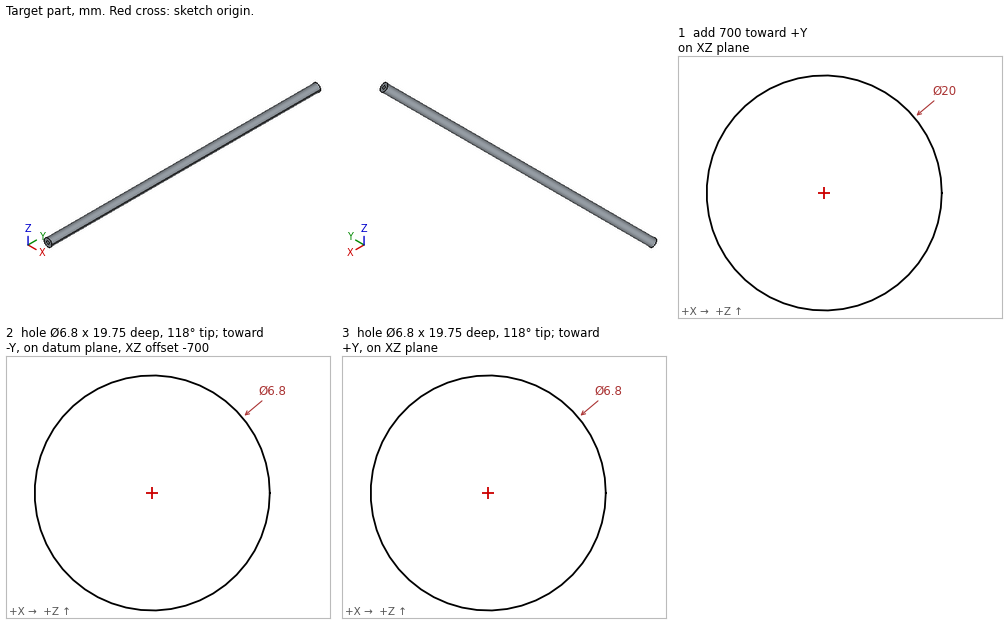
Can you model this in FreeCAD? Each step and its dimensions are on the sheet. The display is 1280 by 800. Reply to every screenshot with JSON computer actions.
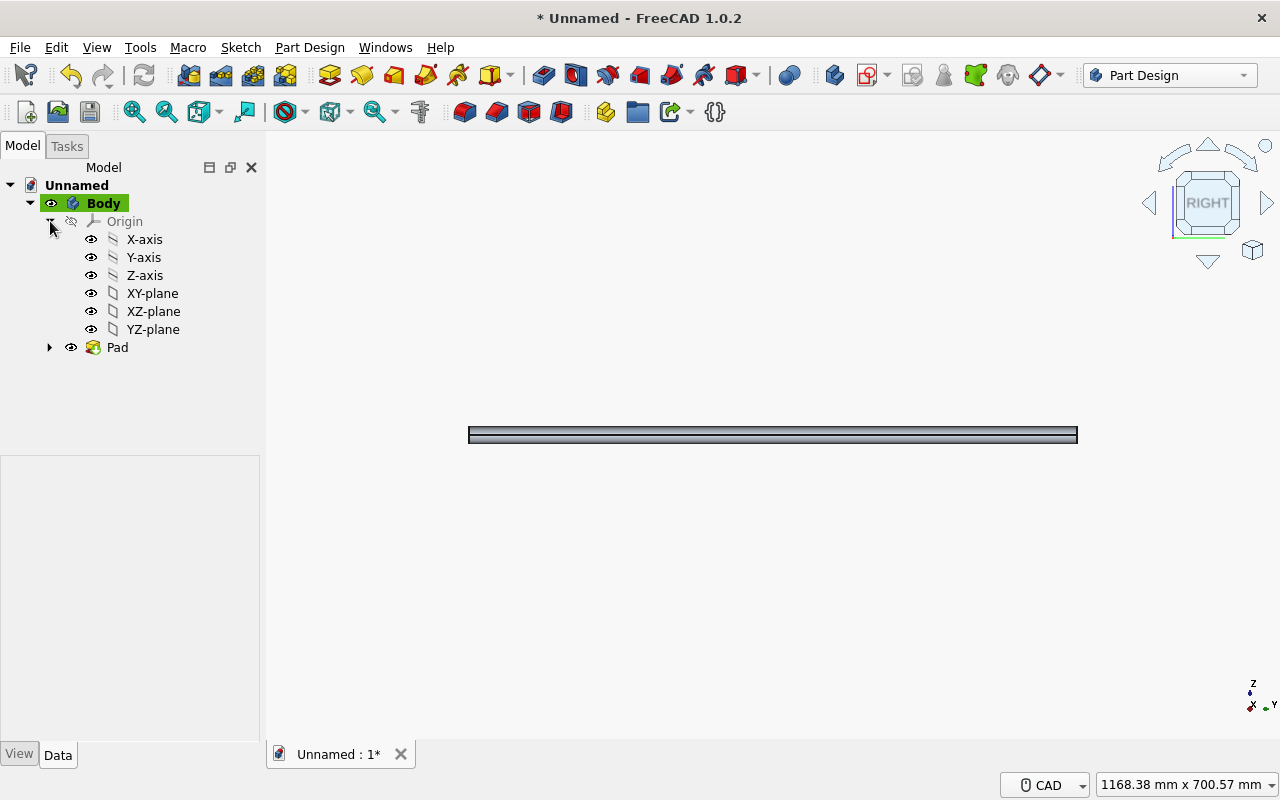
{"action": "left_click", "coordinate": [136, 311]}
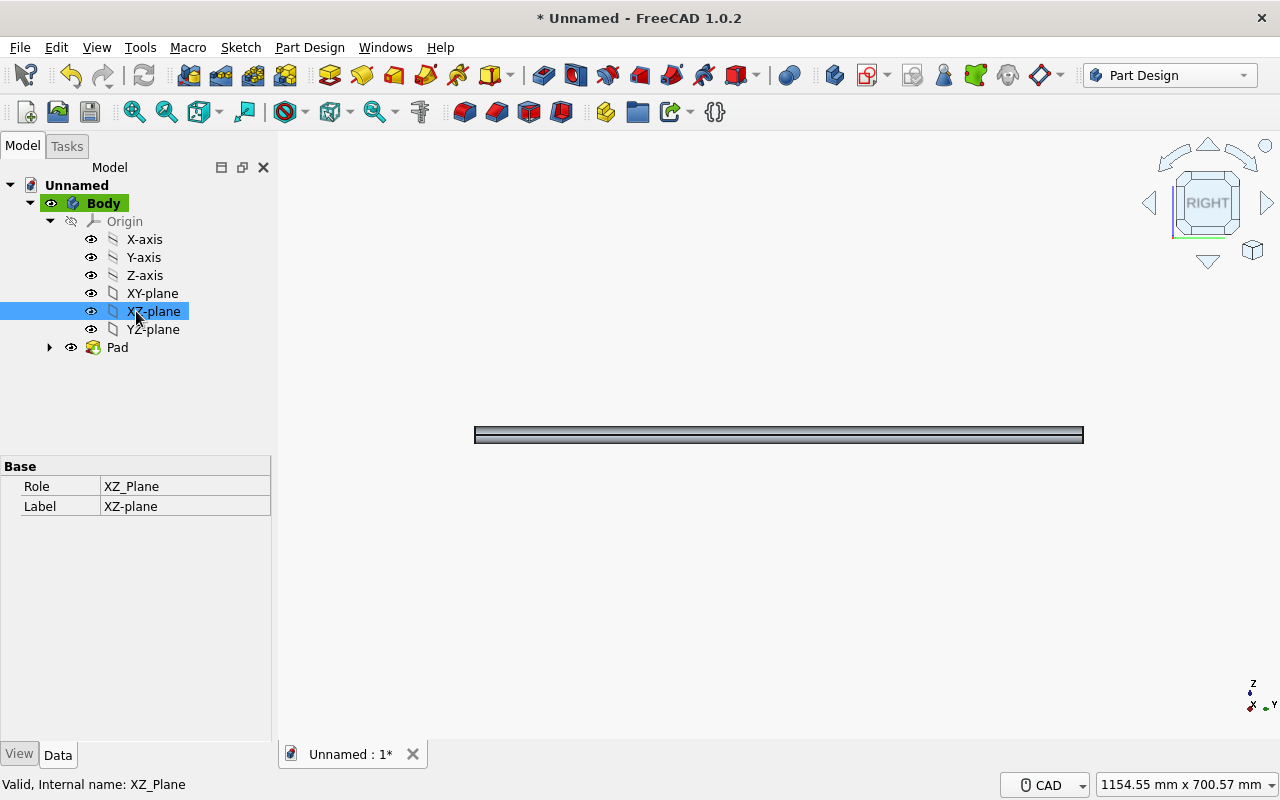
{"action": "left_click", "coordinate": [1040, 76]}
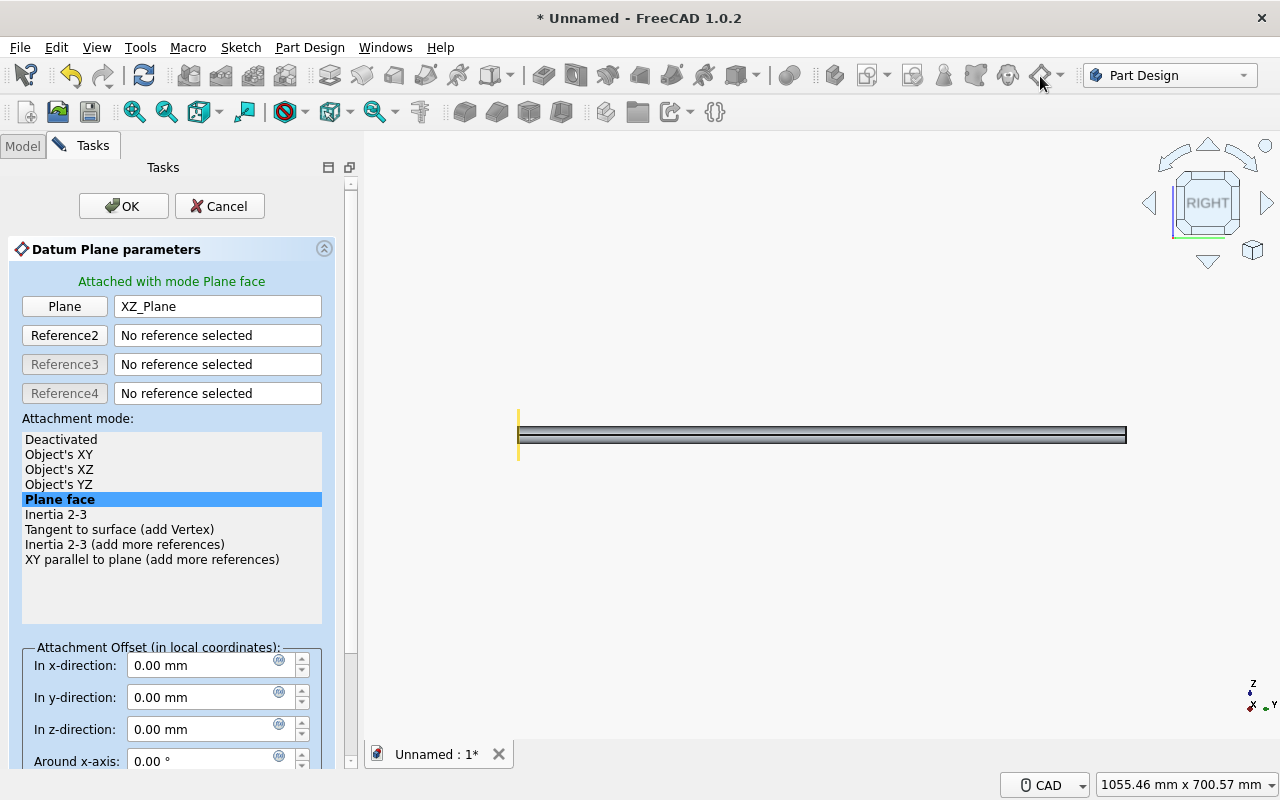
{"action": "triple_click", "coordinate": [210, 729]}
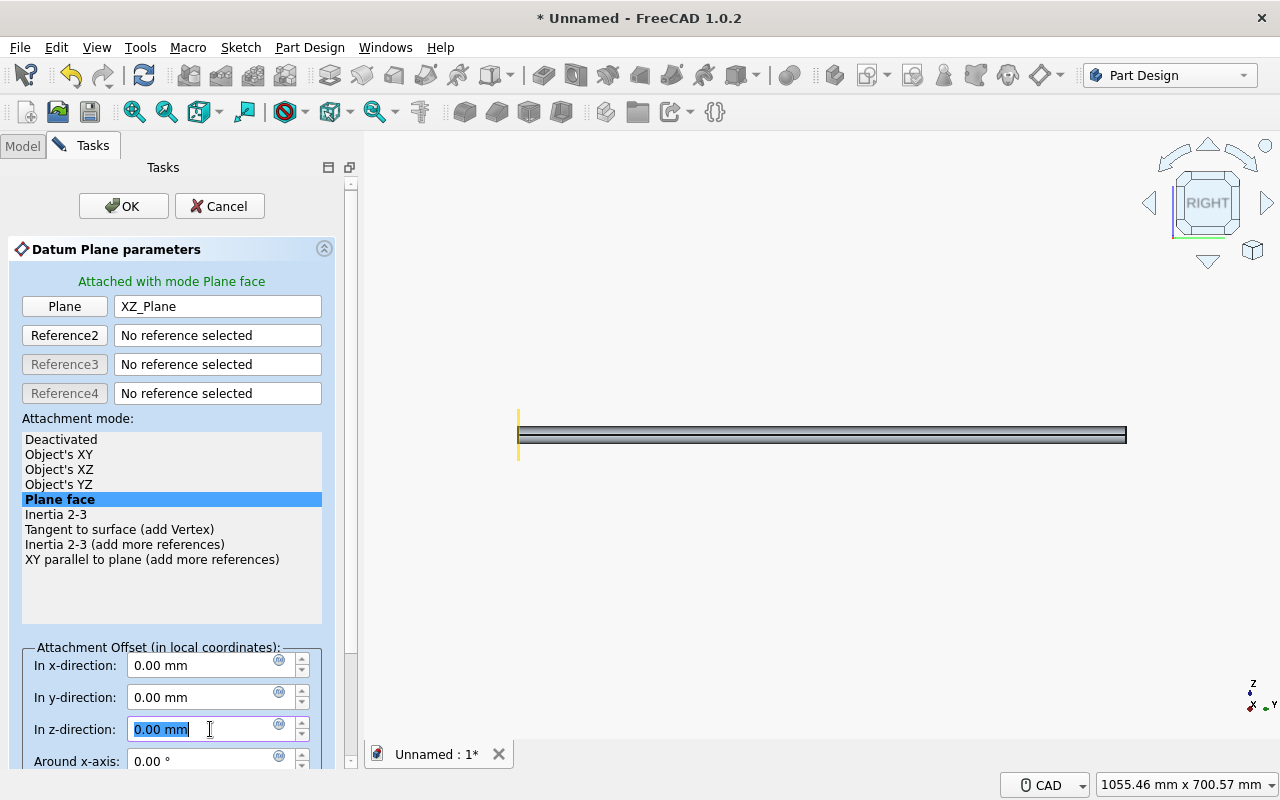
{"action": "type", "text": "-700"}
{"action": "key", "text": "Tab"}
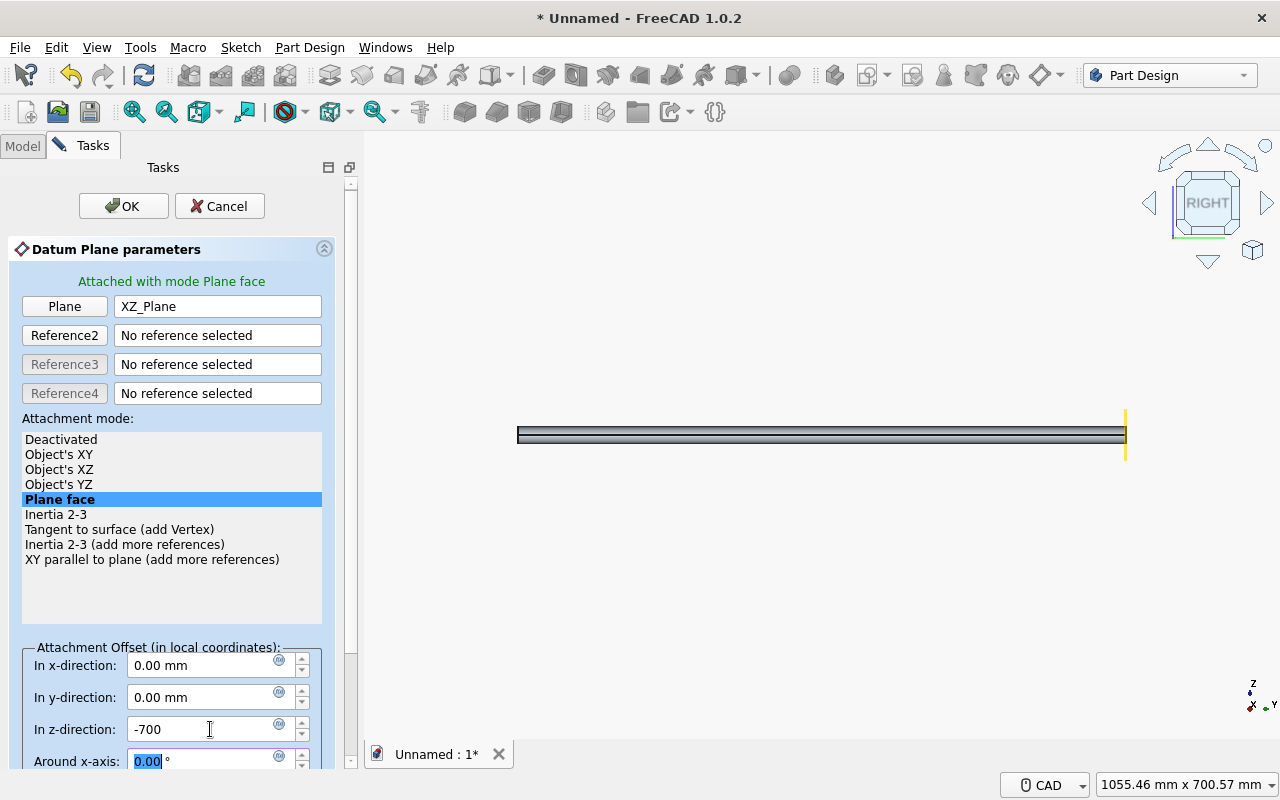
{"action": "left_click", "coordinate": [124, 206]}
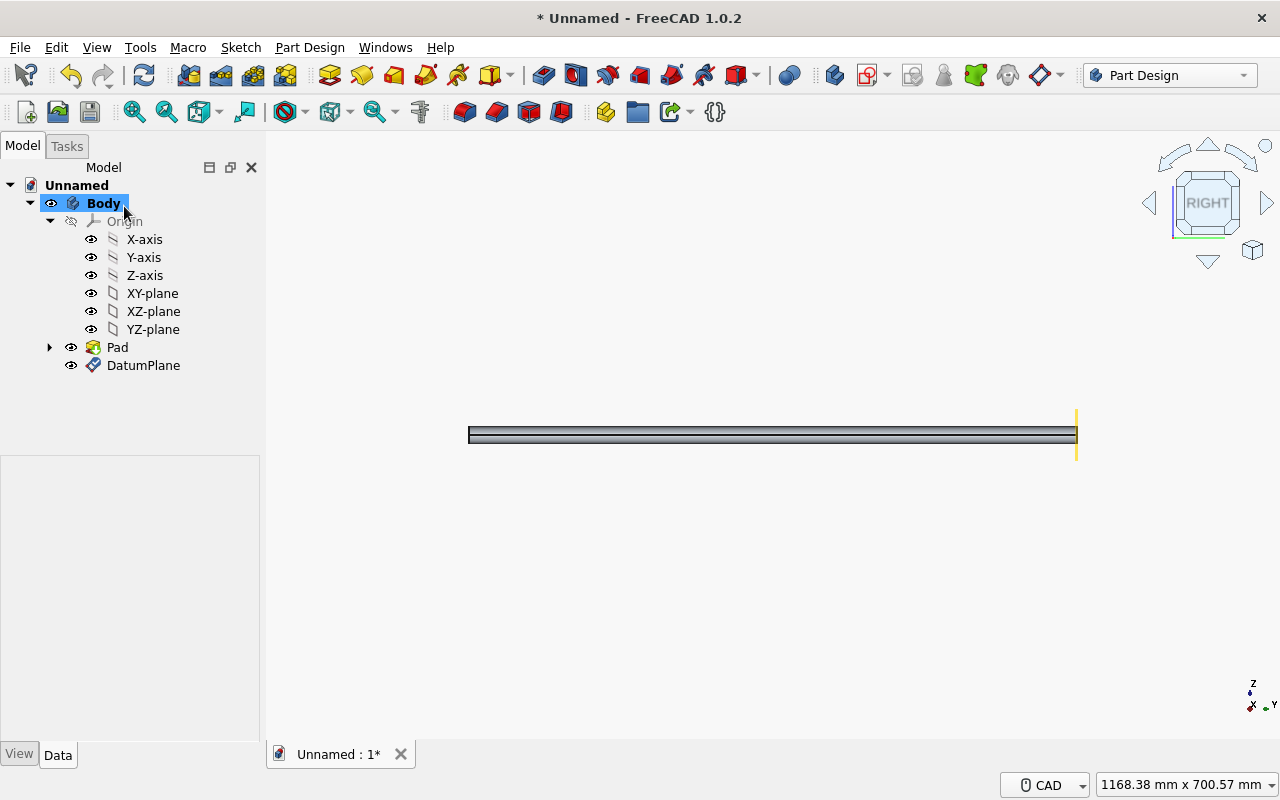
{"action": "left_click", "coordinate": [116, 365]}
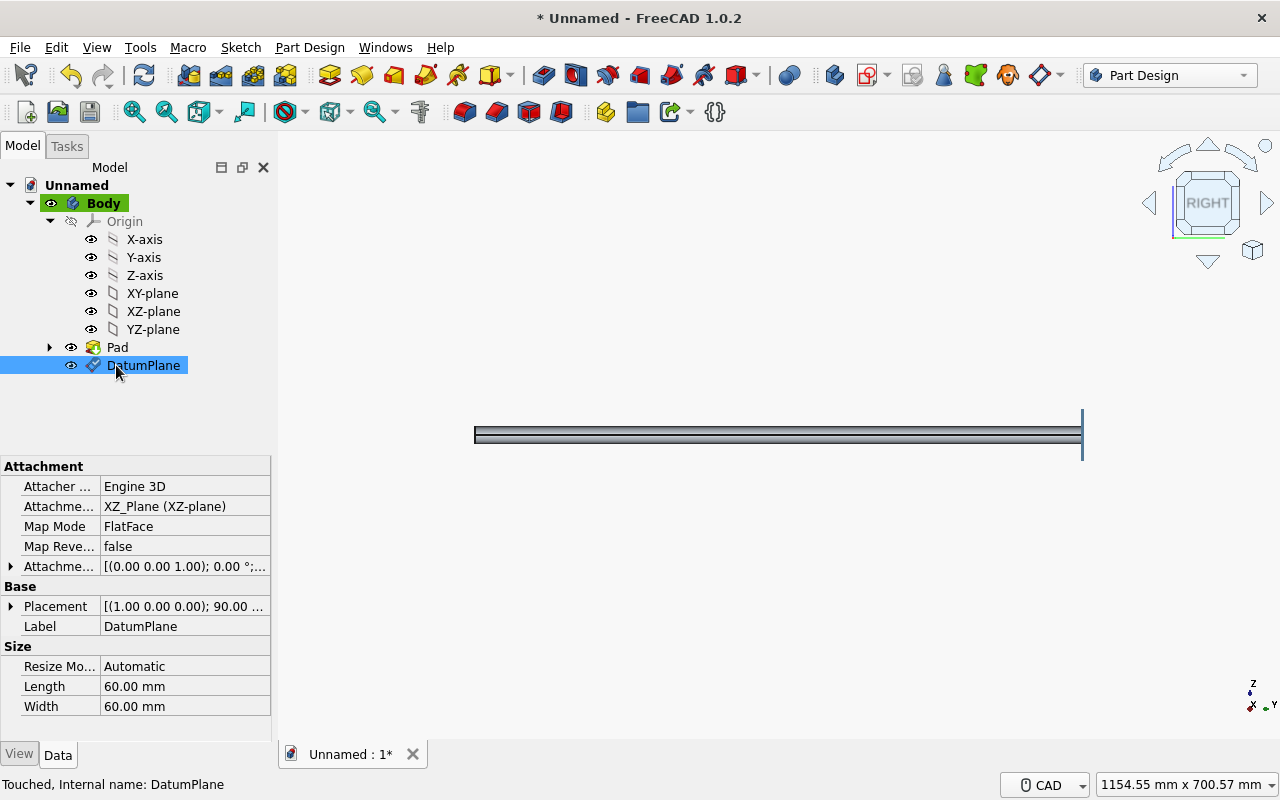
{"action": "left_click", "coordinate": [868, 76]}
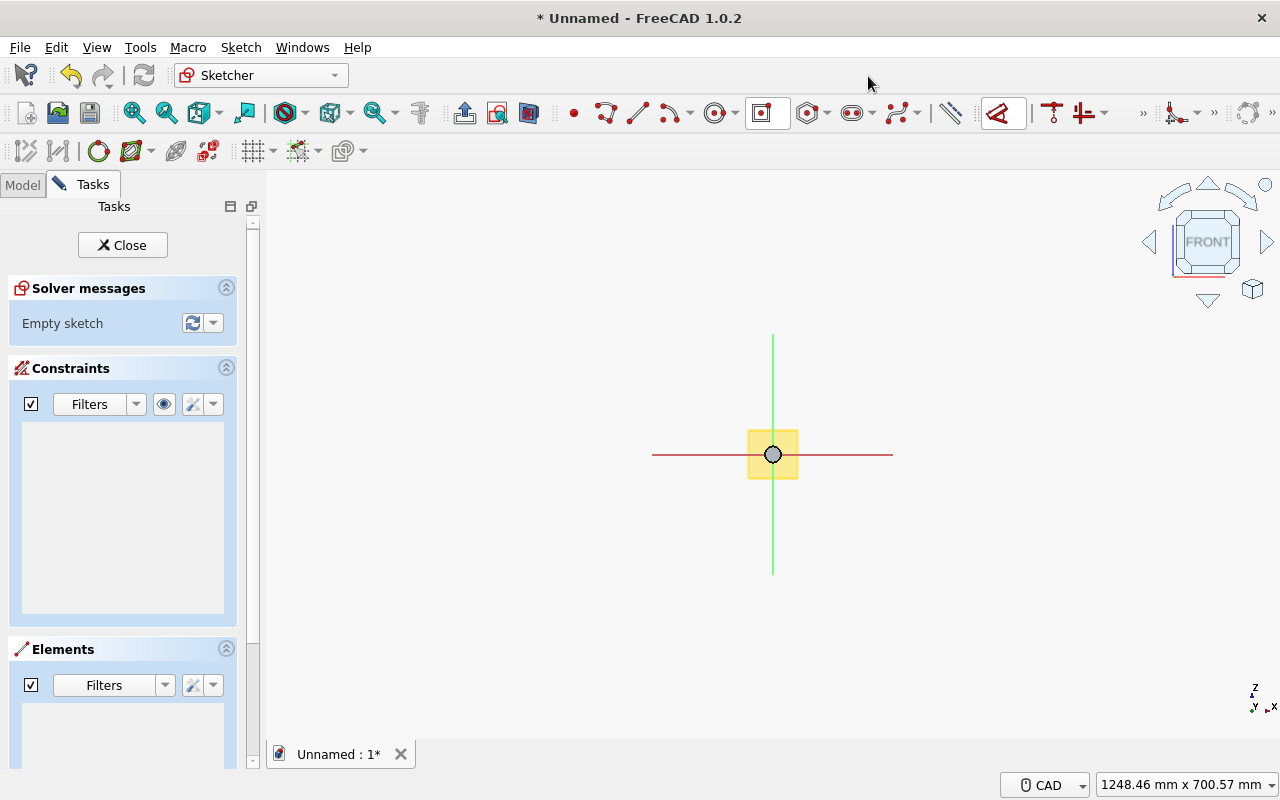
{"action": "left_click", "coordinate": [530, 114]}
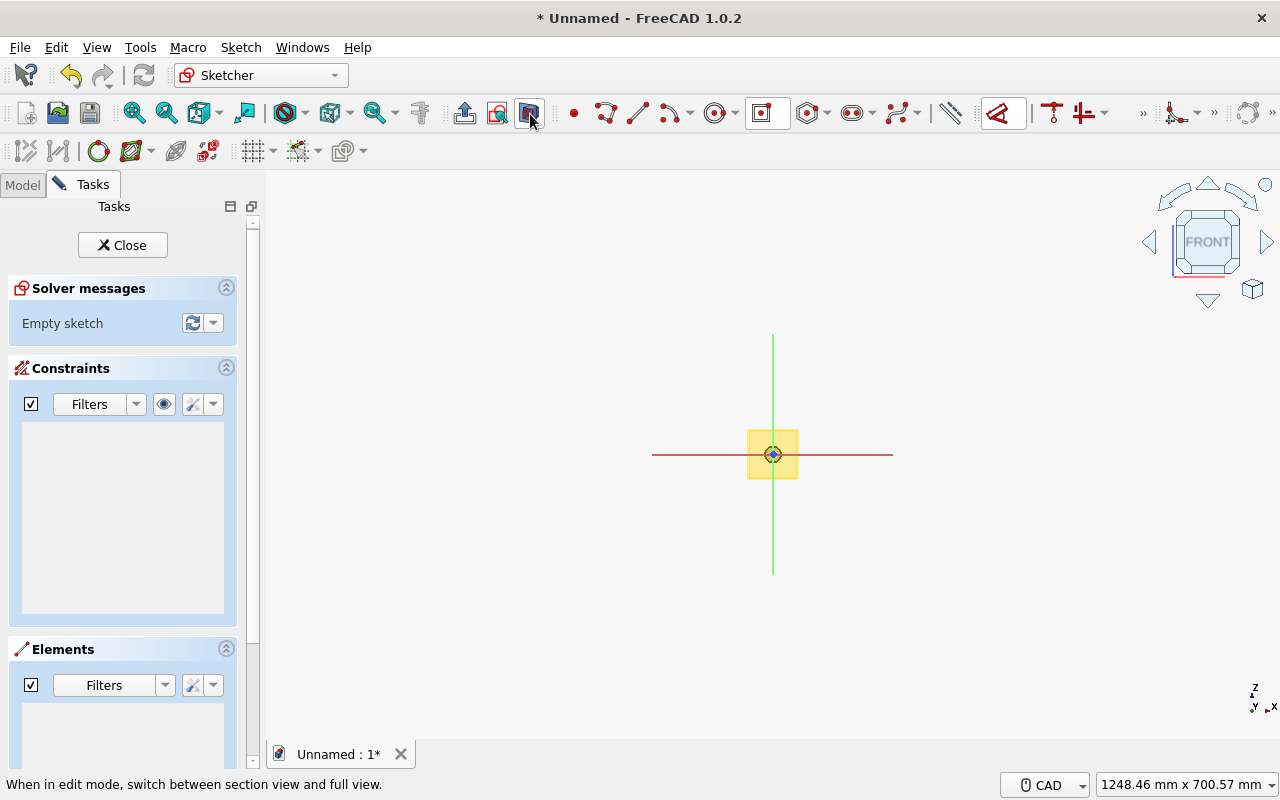
{"action": "scroll", "coordinate": [777, 455], "scroll_direction": "up", "scroll_amount": 15}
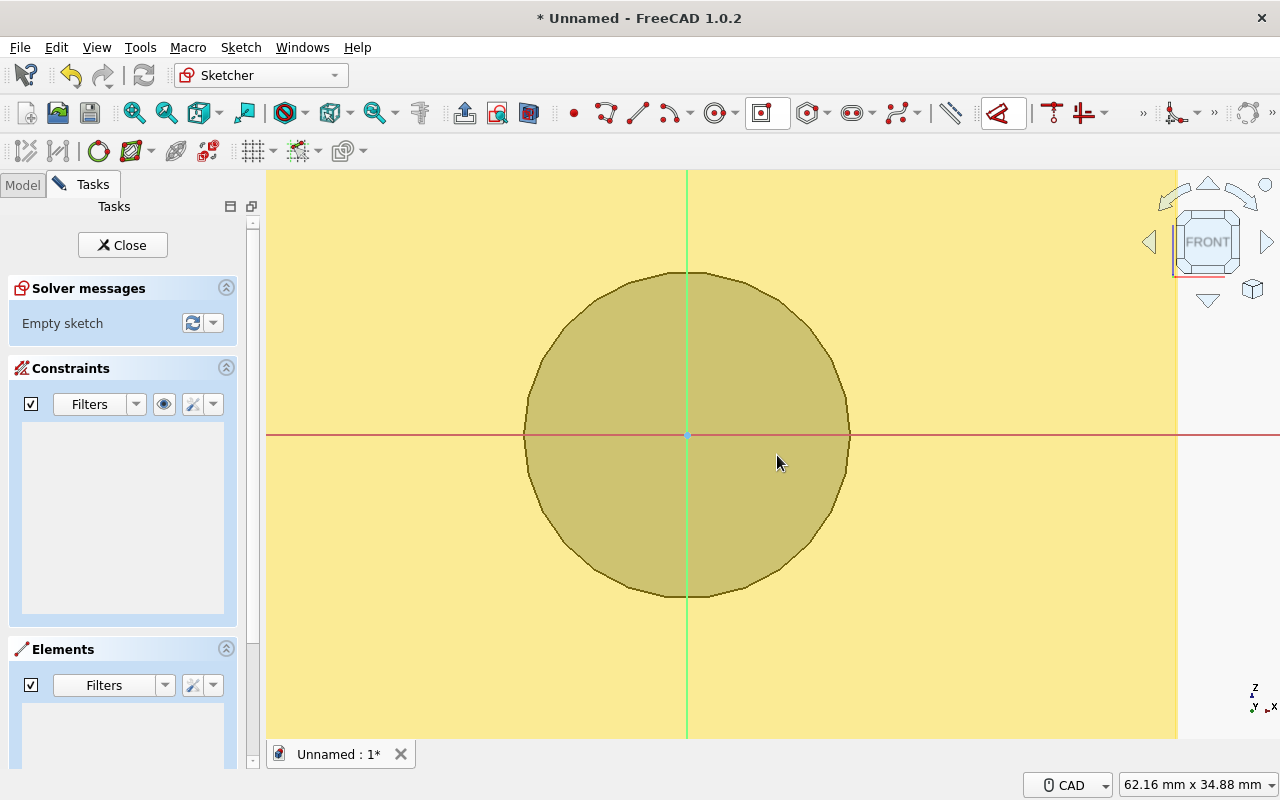
{"action": "scroll", "coordinate": [680, 427], "scroll_direction": "up", "scroll_amount": 6}